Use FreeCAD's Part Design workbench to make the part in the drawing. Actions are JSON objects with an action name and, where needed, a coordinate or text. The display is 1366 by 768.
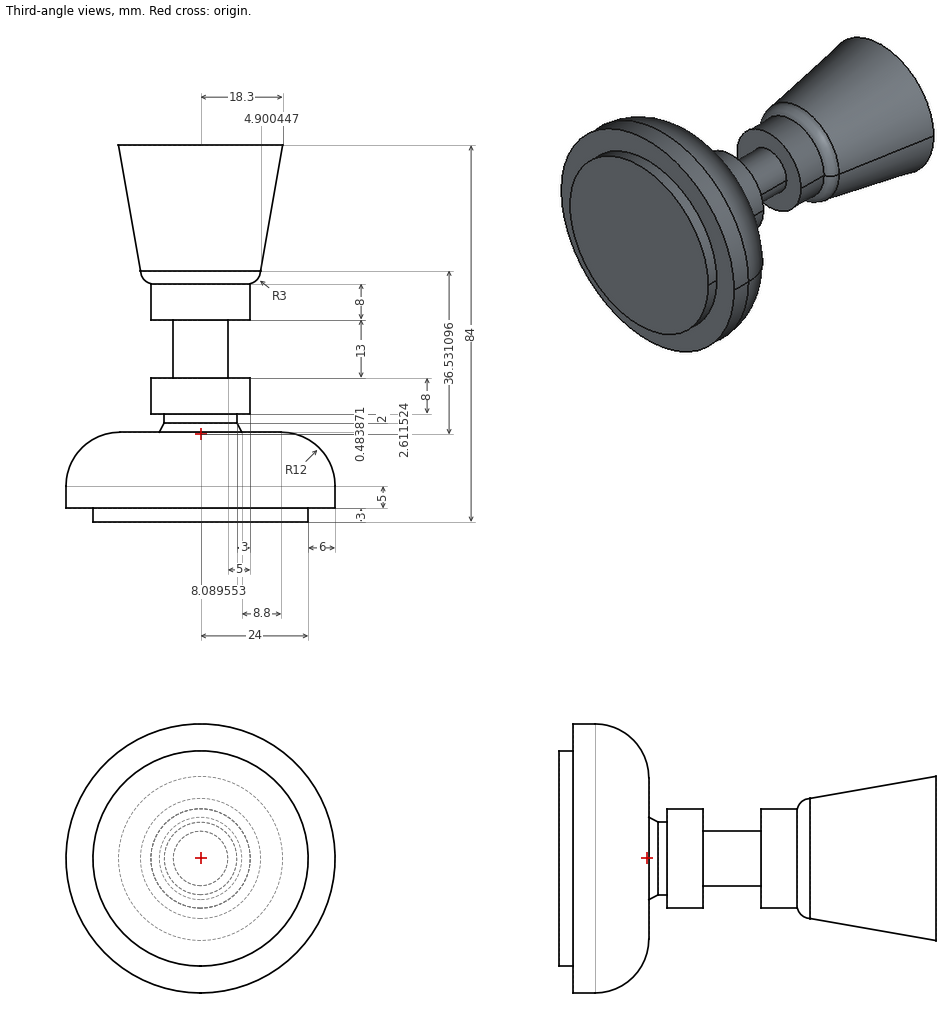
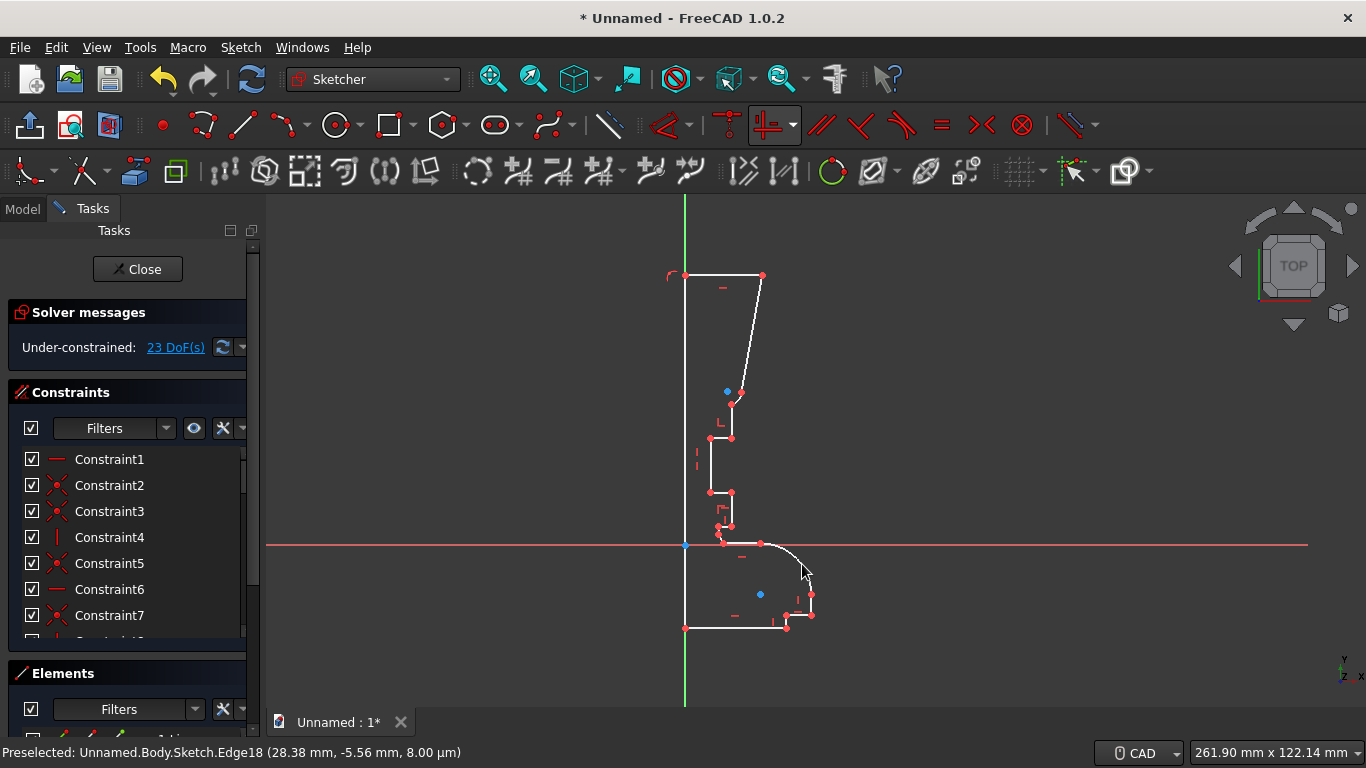
{"action": "scroll", "coordinate": [750, 543], "scroll_direction": "up", "scroll_amount": 2}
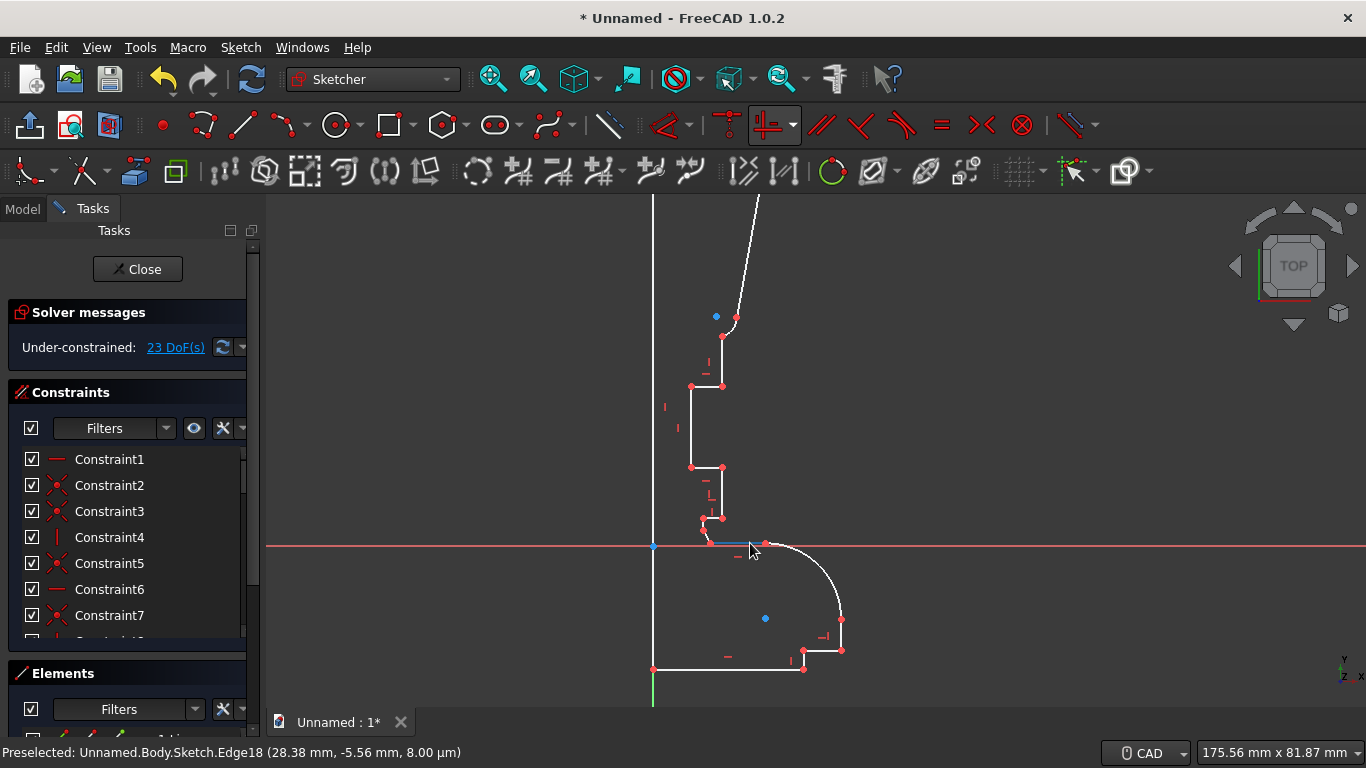
{"action": "left_click", "coordinate": [749, 543]}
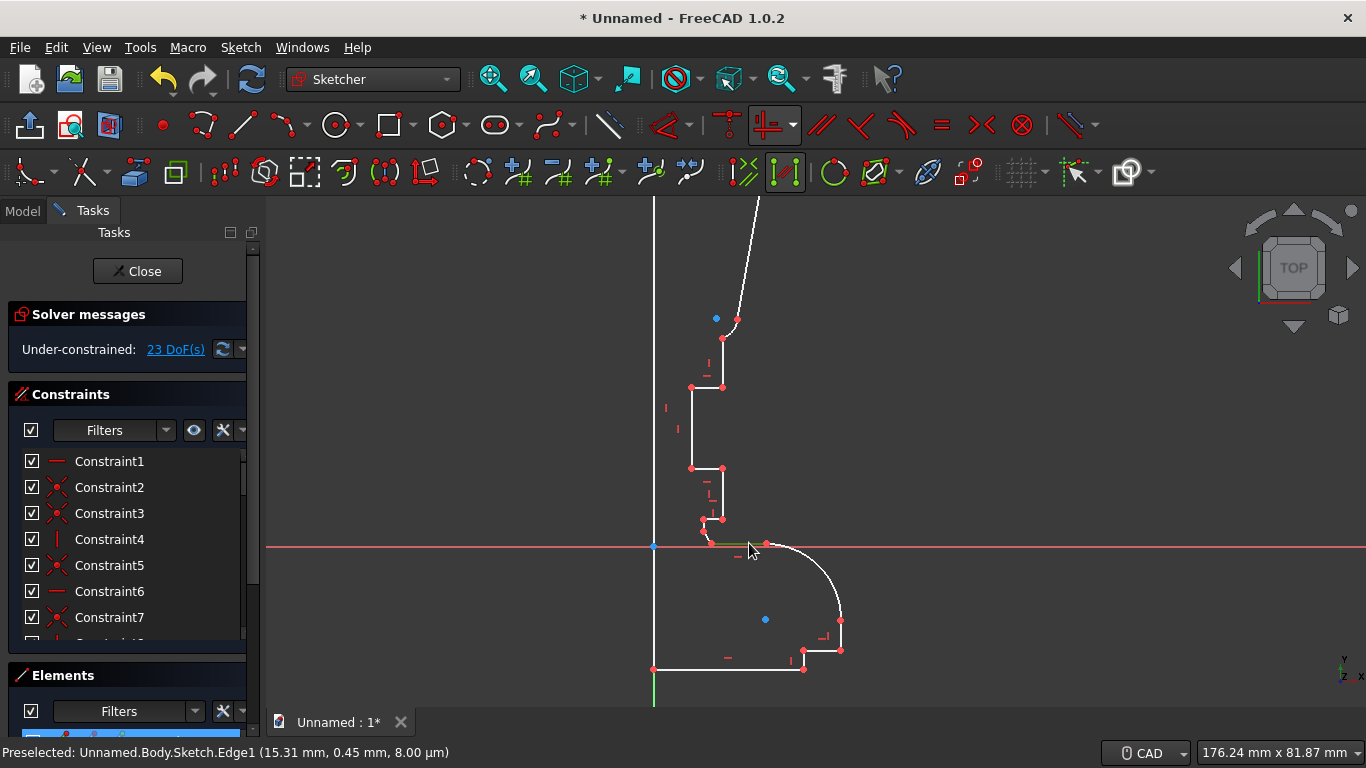
{"action": "left_click", "coordinate": [833, 586]}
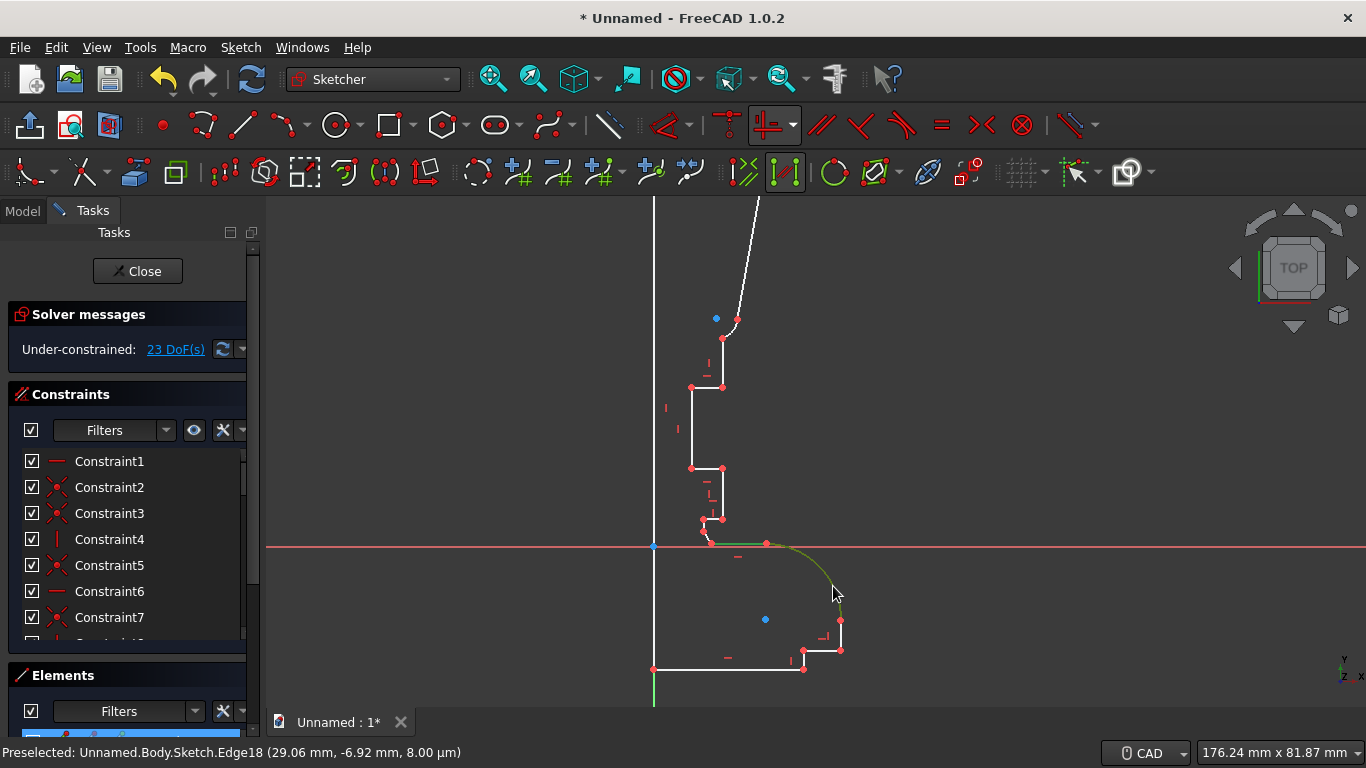
{"action": "key", "text": "t"}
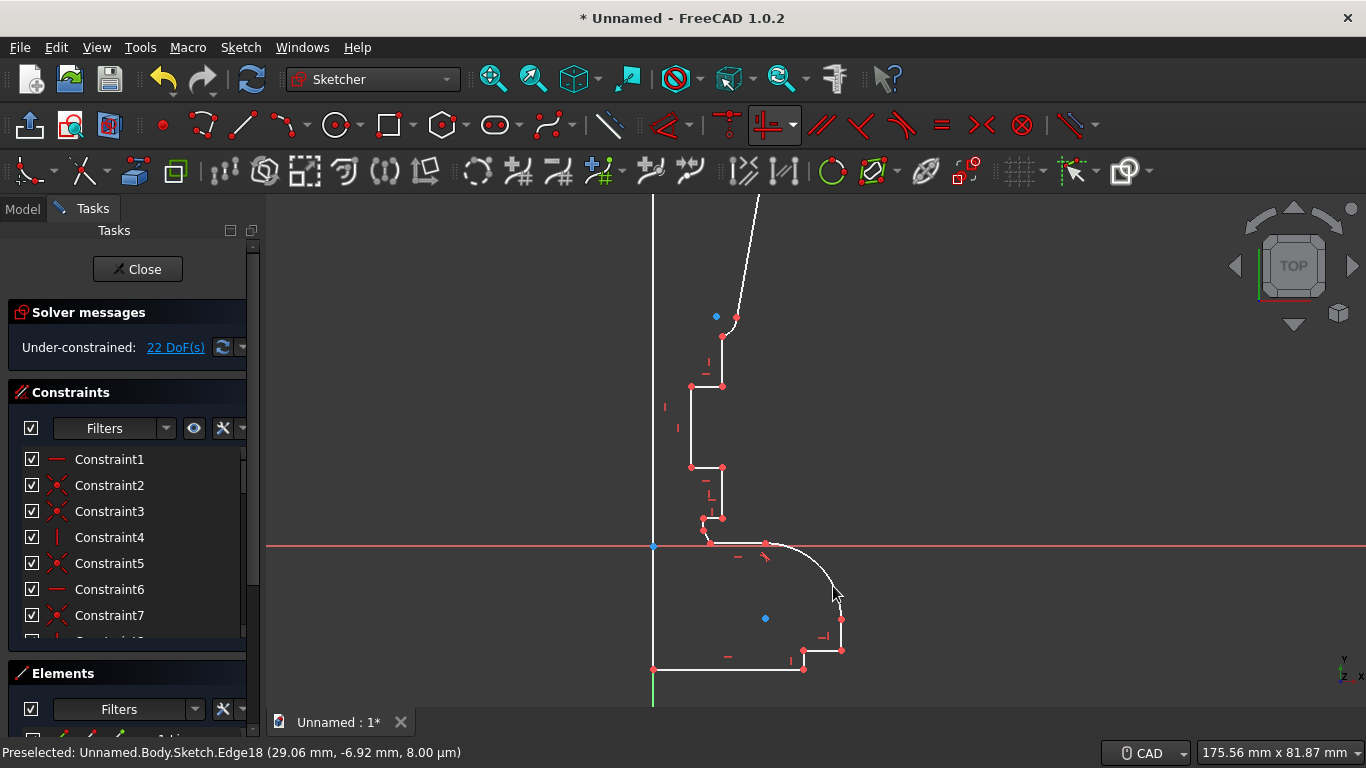
{"action": "scroll", "coordinate": [841, 641], "scroll_direction": "up", "scroll_amount": 2}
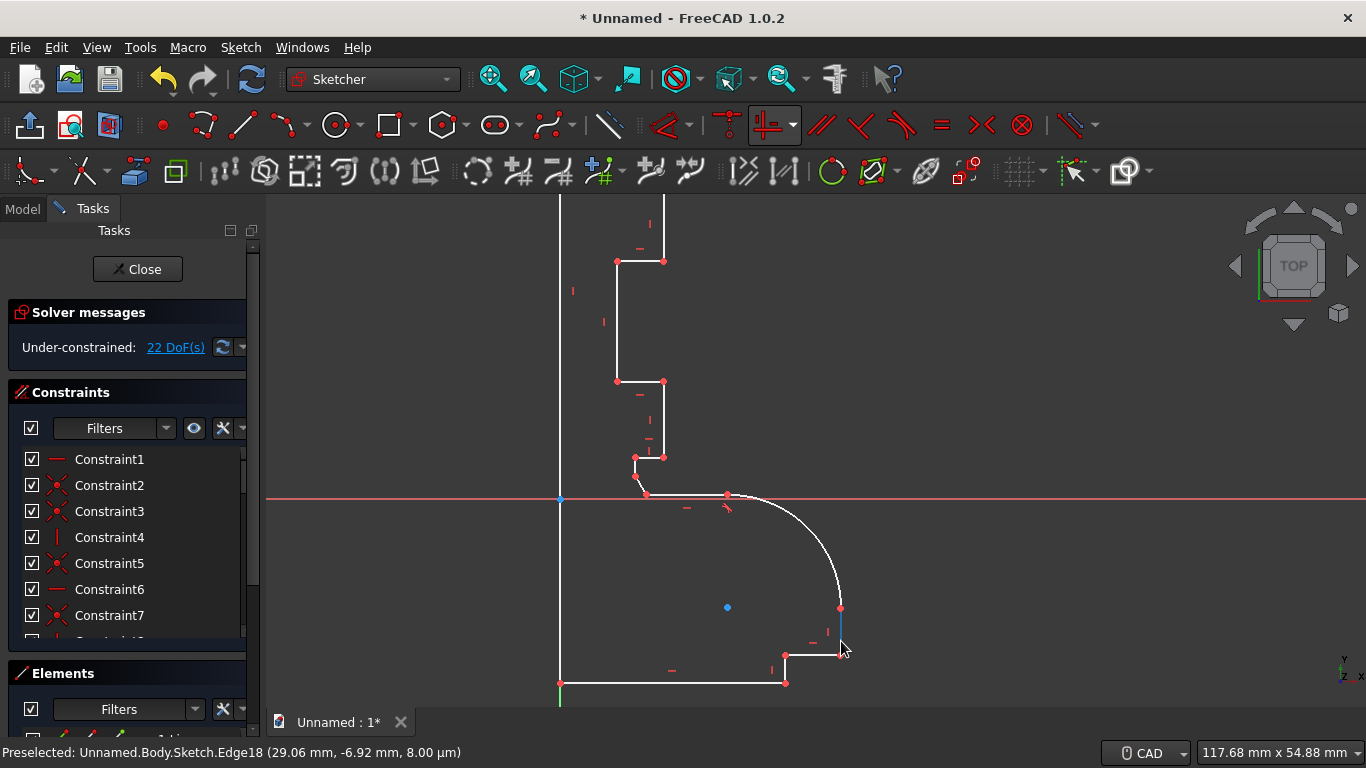
{"action": "left_click", "coordinate": [841, 641]}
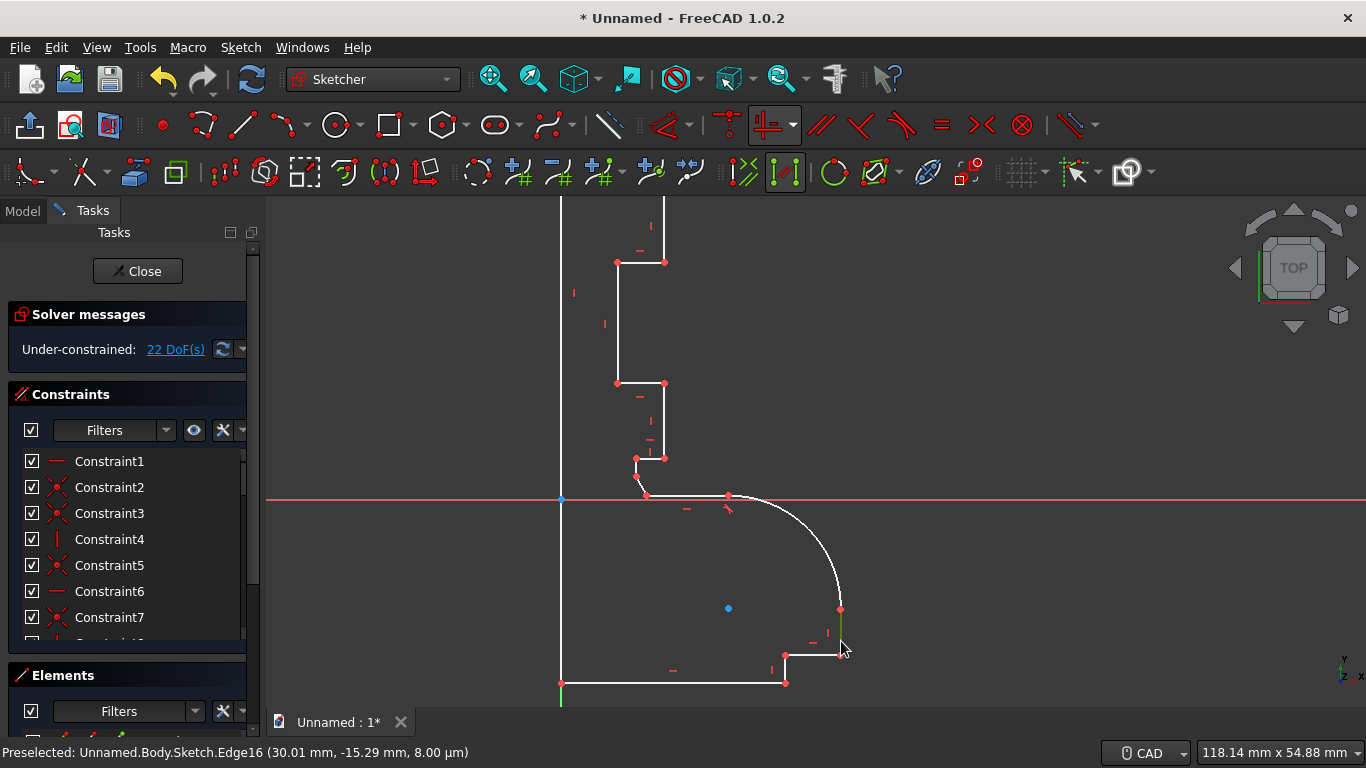
{"action": "left_click", "coordinate": [829, 558]}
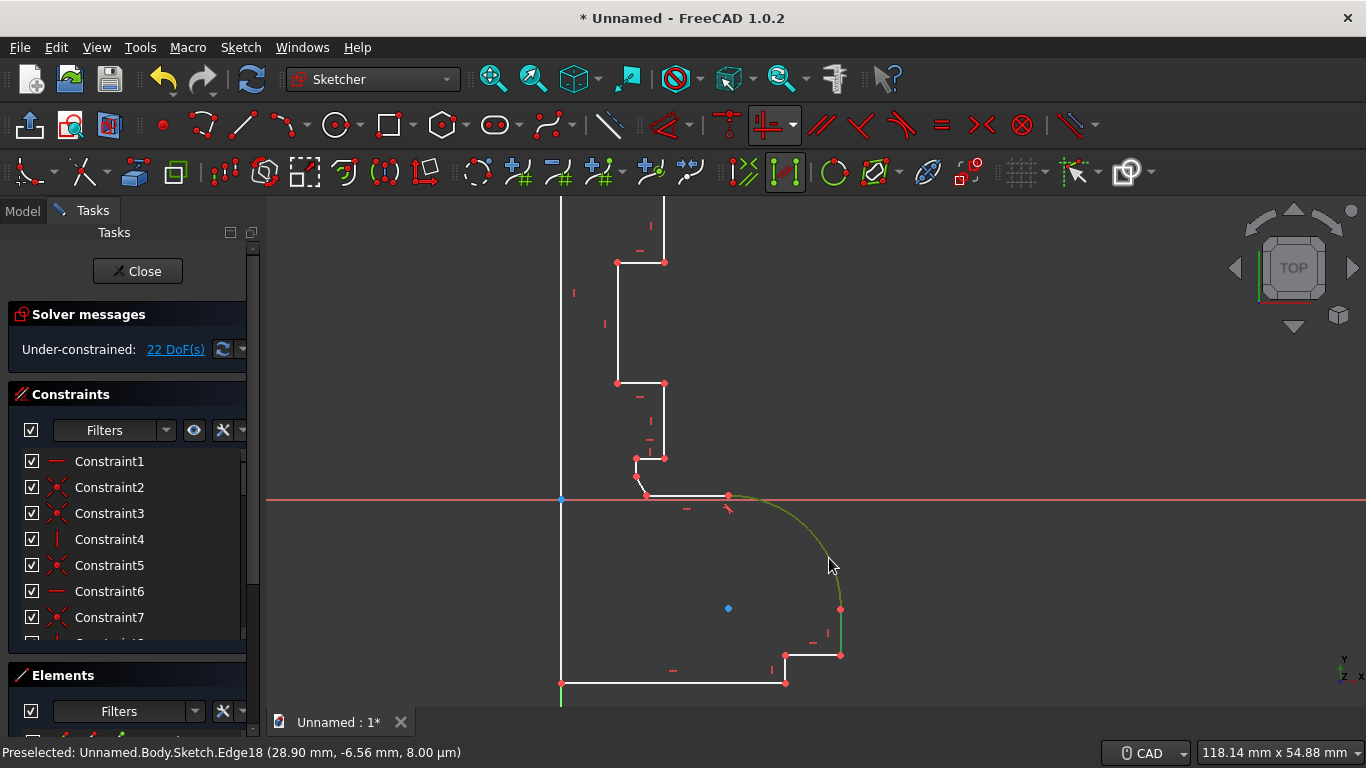
{"action": "left_click", "coordinate": [902, 126]}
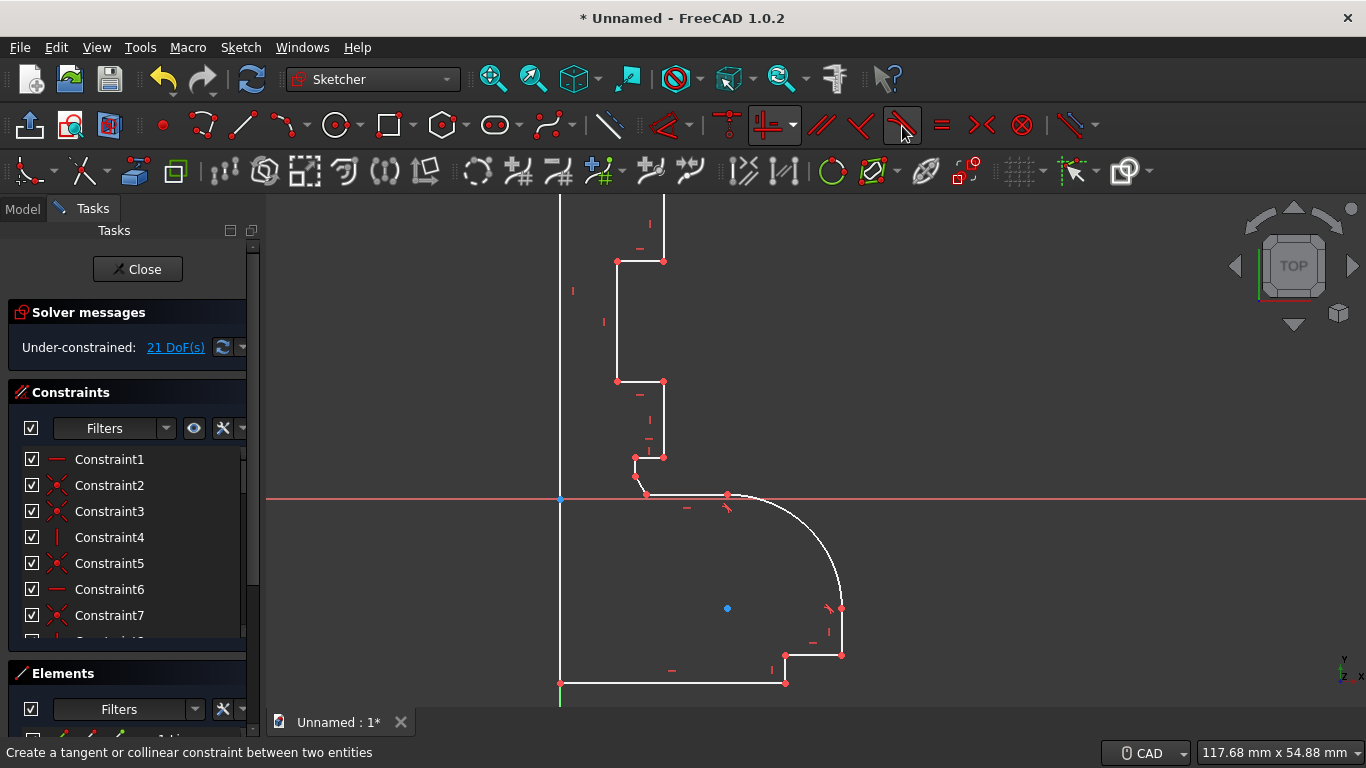
{"action": "left_click", "coordinate": [664, 126]}